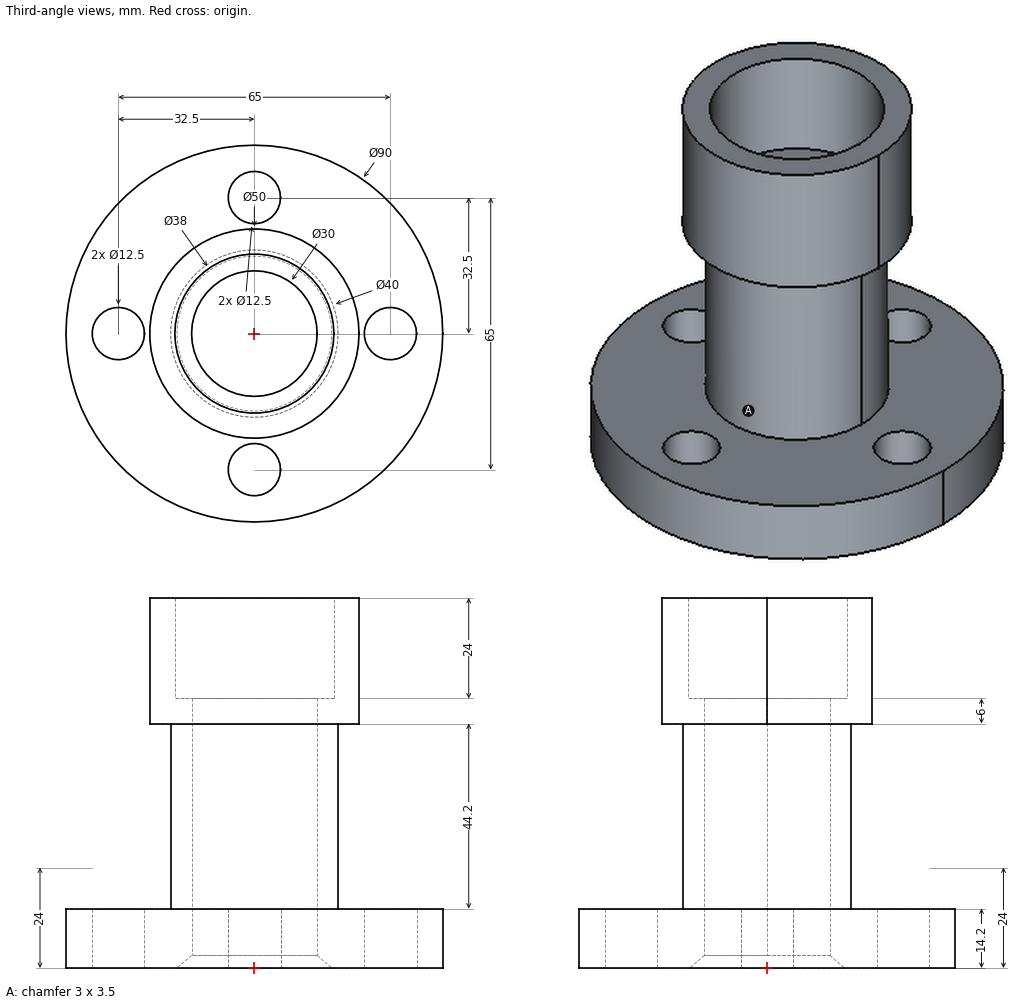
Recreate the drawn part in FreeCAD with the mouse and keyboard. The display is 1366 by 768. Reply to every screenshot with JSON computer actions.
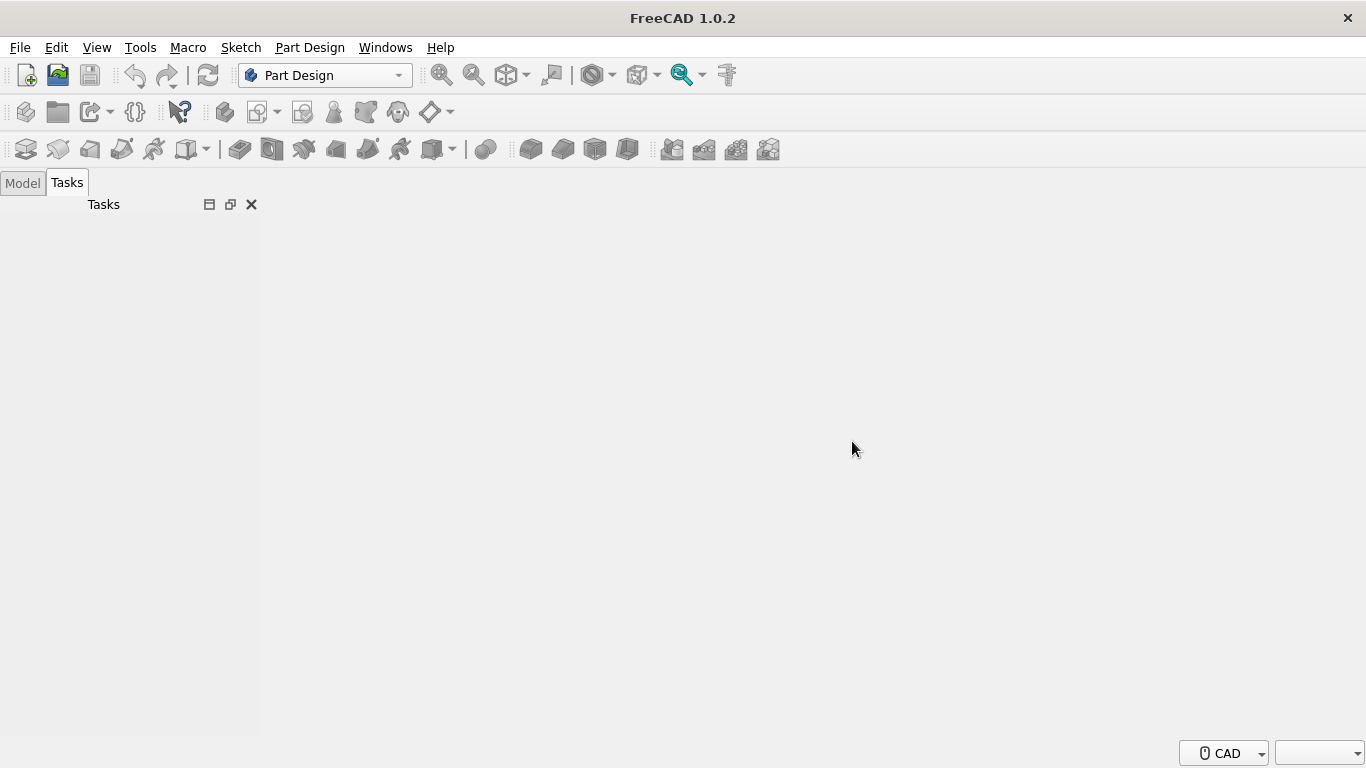
{"action": "left_click", "coordinate": [26, 76]}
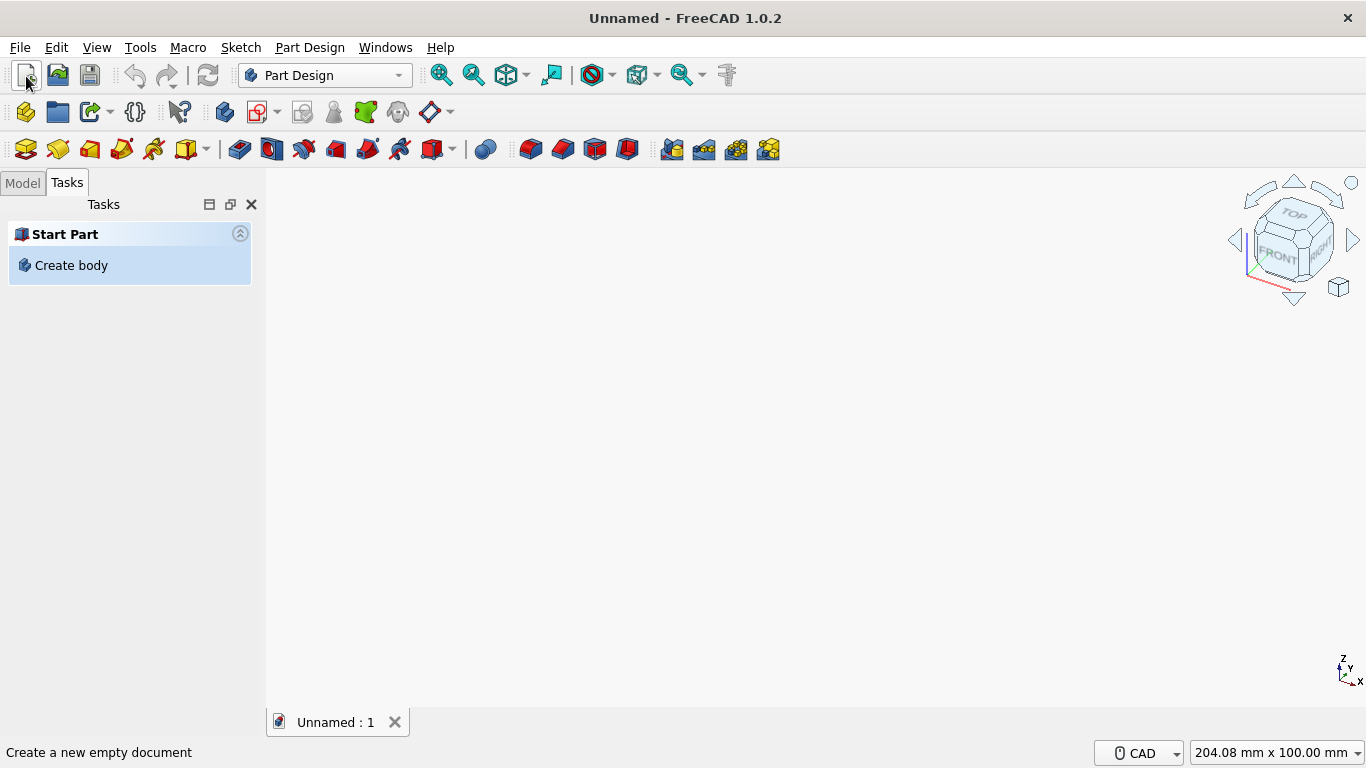
{"action": "left_click", "coordinate": [258, 112]}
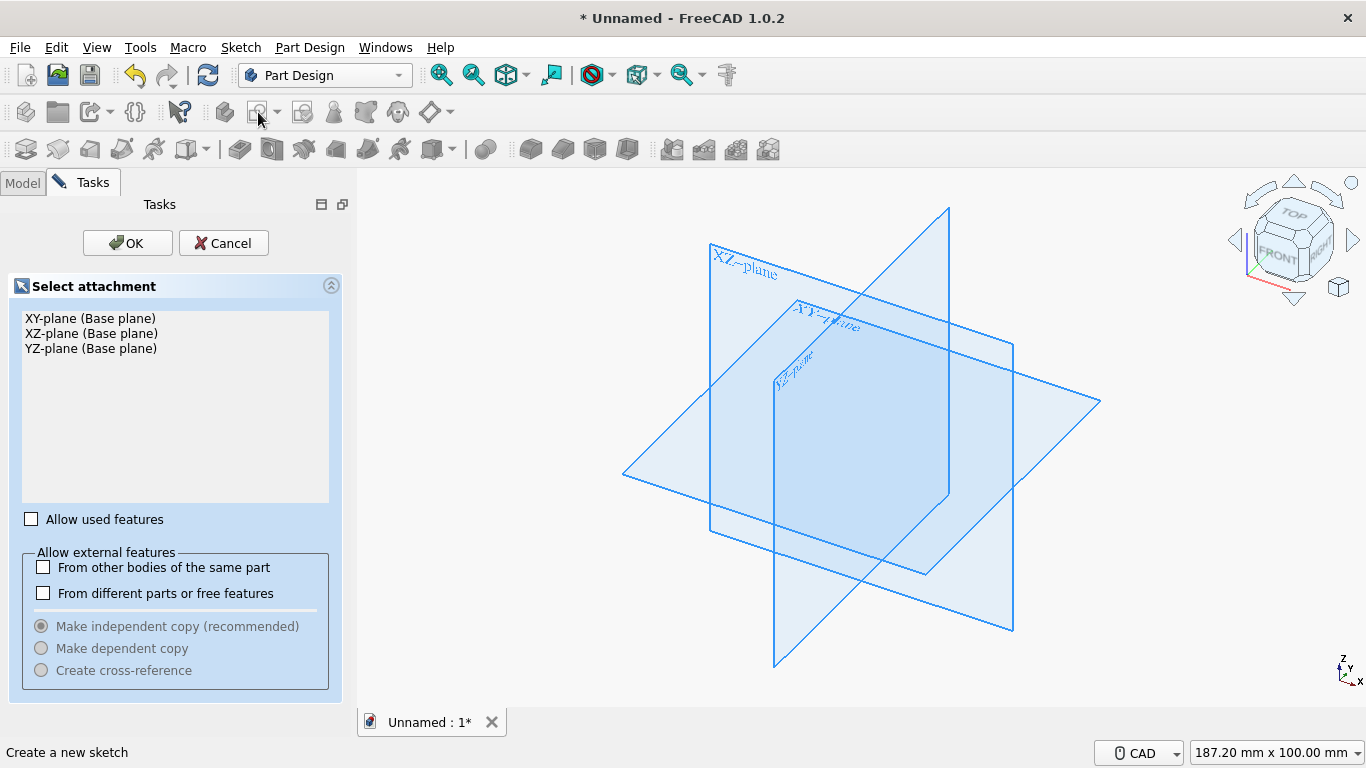
{"action": "left_click", "coordinate": [82, 318]}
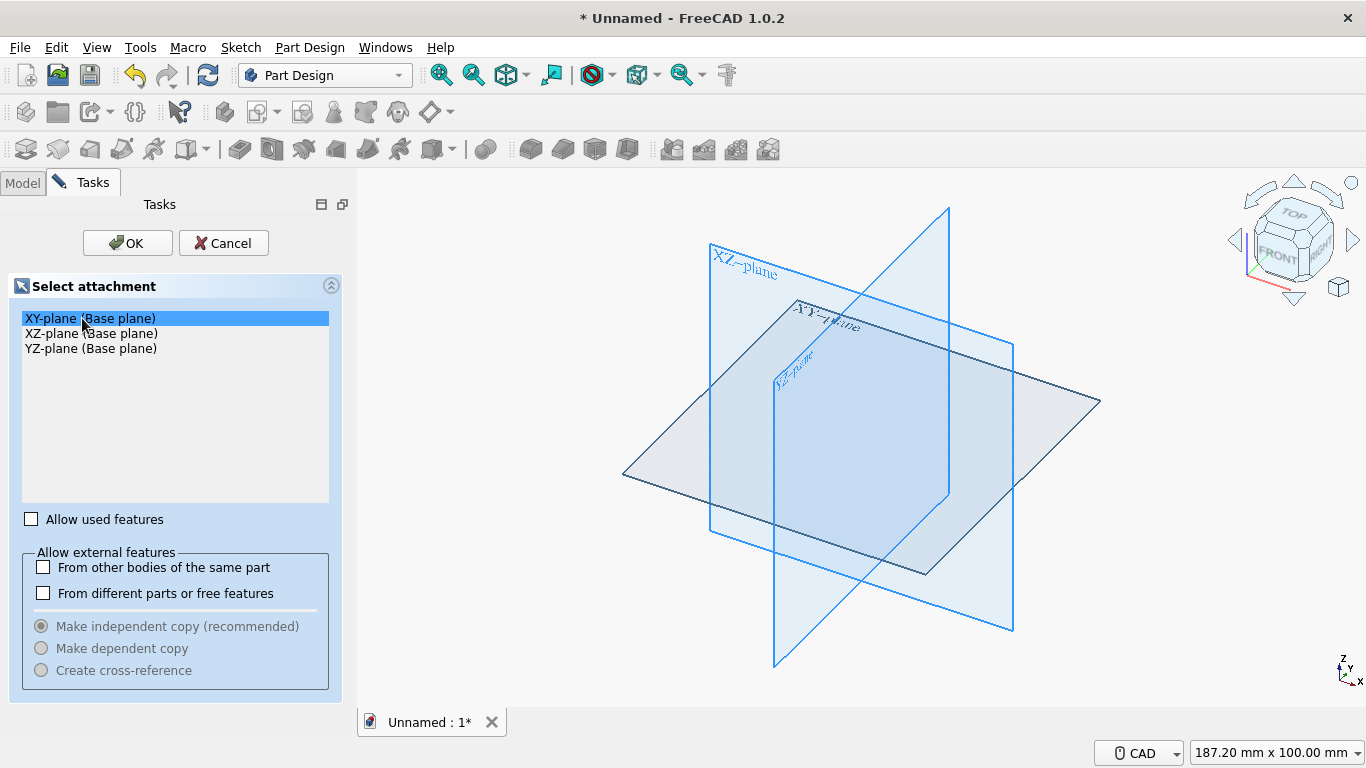
{"action": "left_click", "coordinate": [128, 243]}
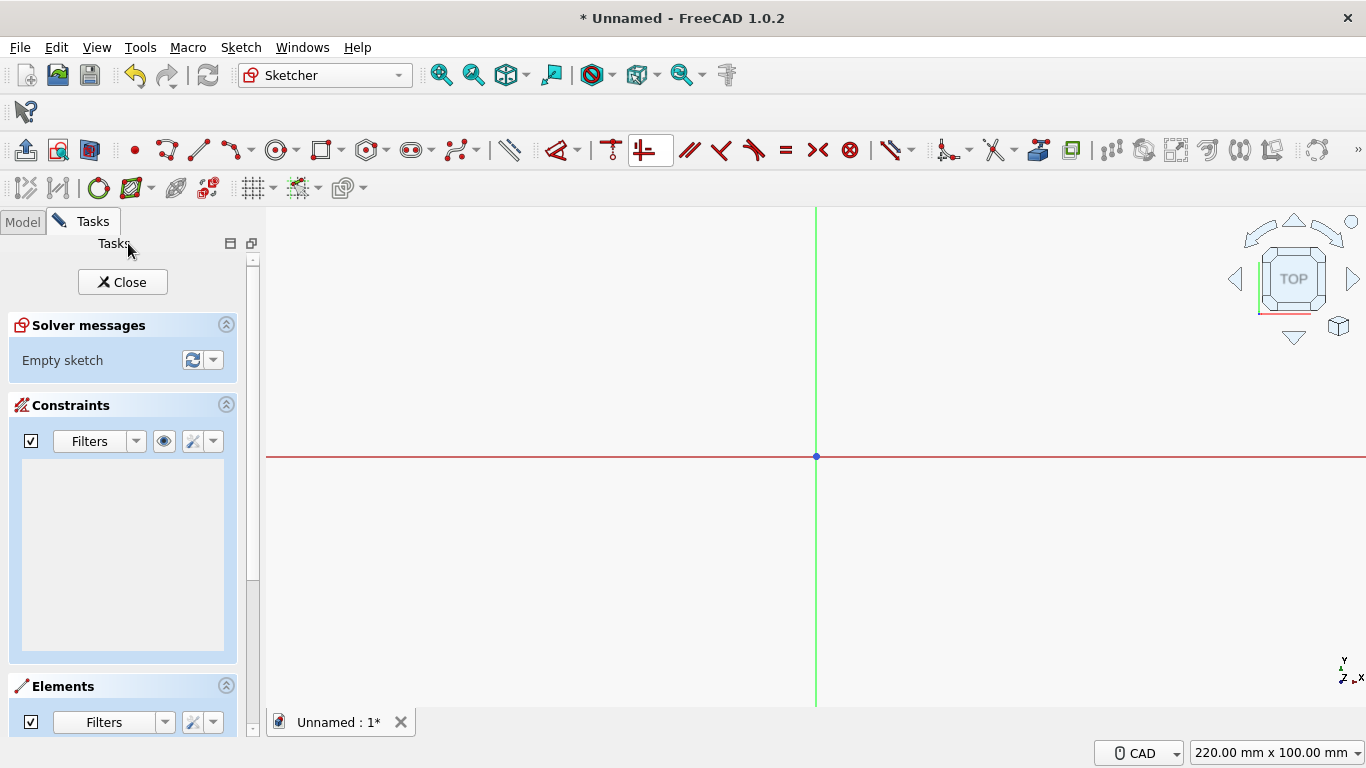
{"action": "scroll", "coordinate": [608, 457], "scroll_direction": "down", "scroll_amount": 2}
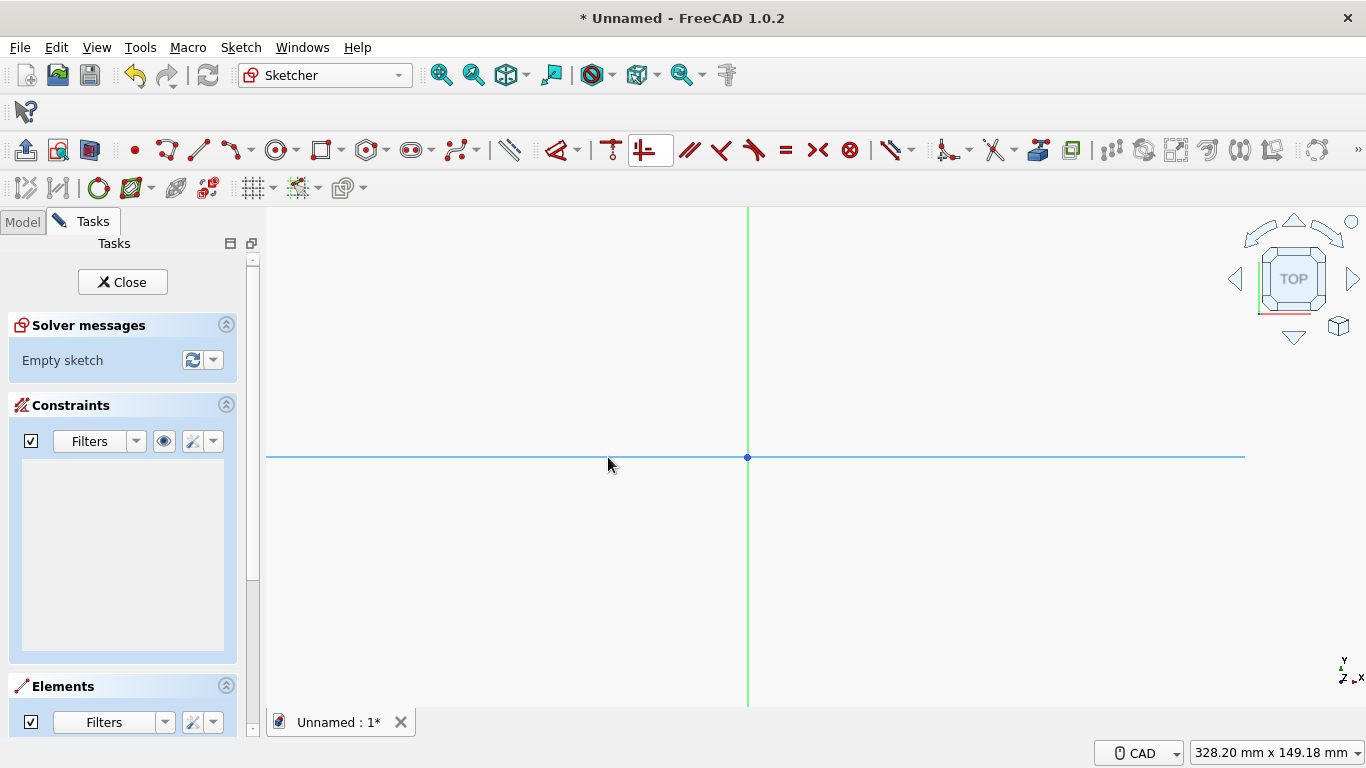
{"action": "left_click", "coordinate": [276, 150]}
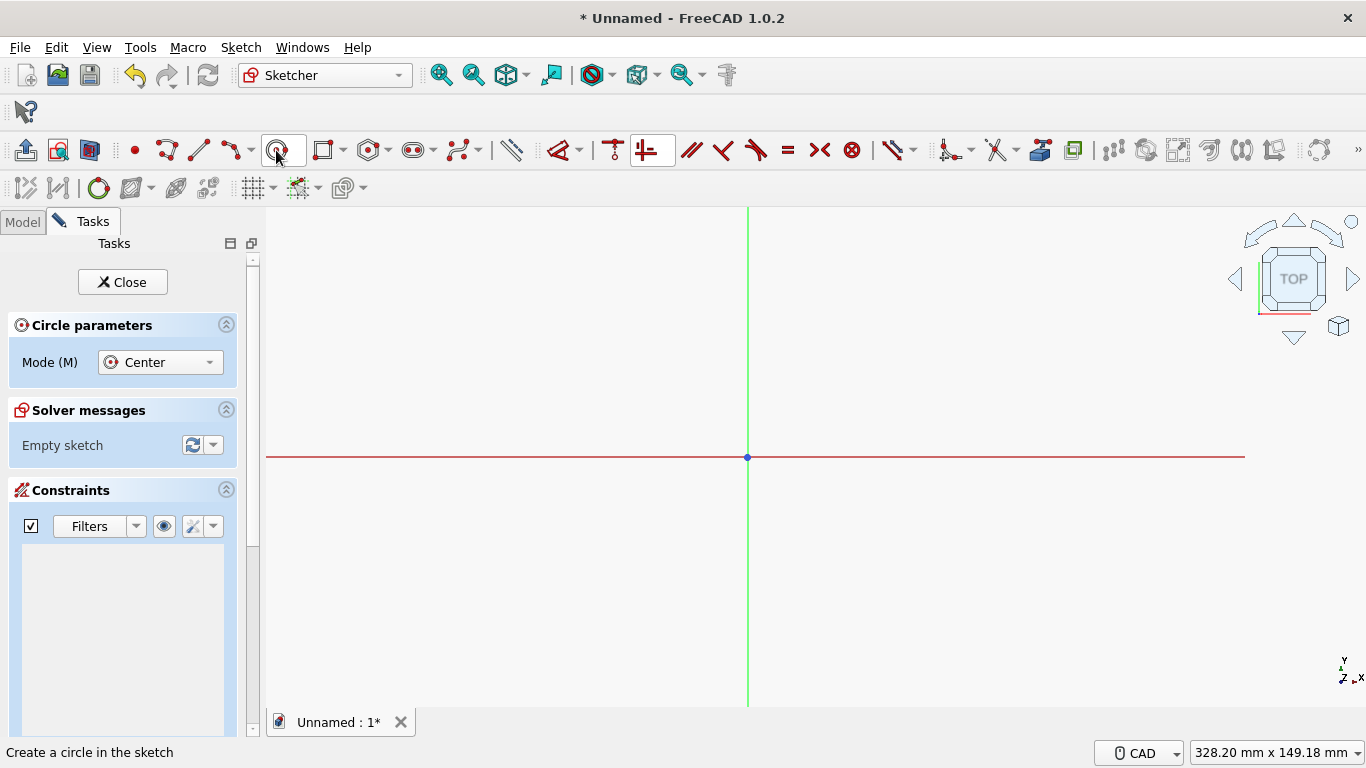
{"action": "left_click", "coordinate": [748, 457]}
{"action": "mouse_move", "coordinate": [854, 351]}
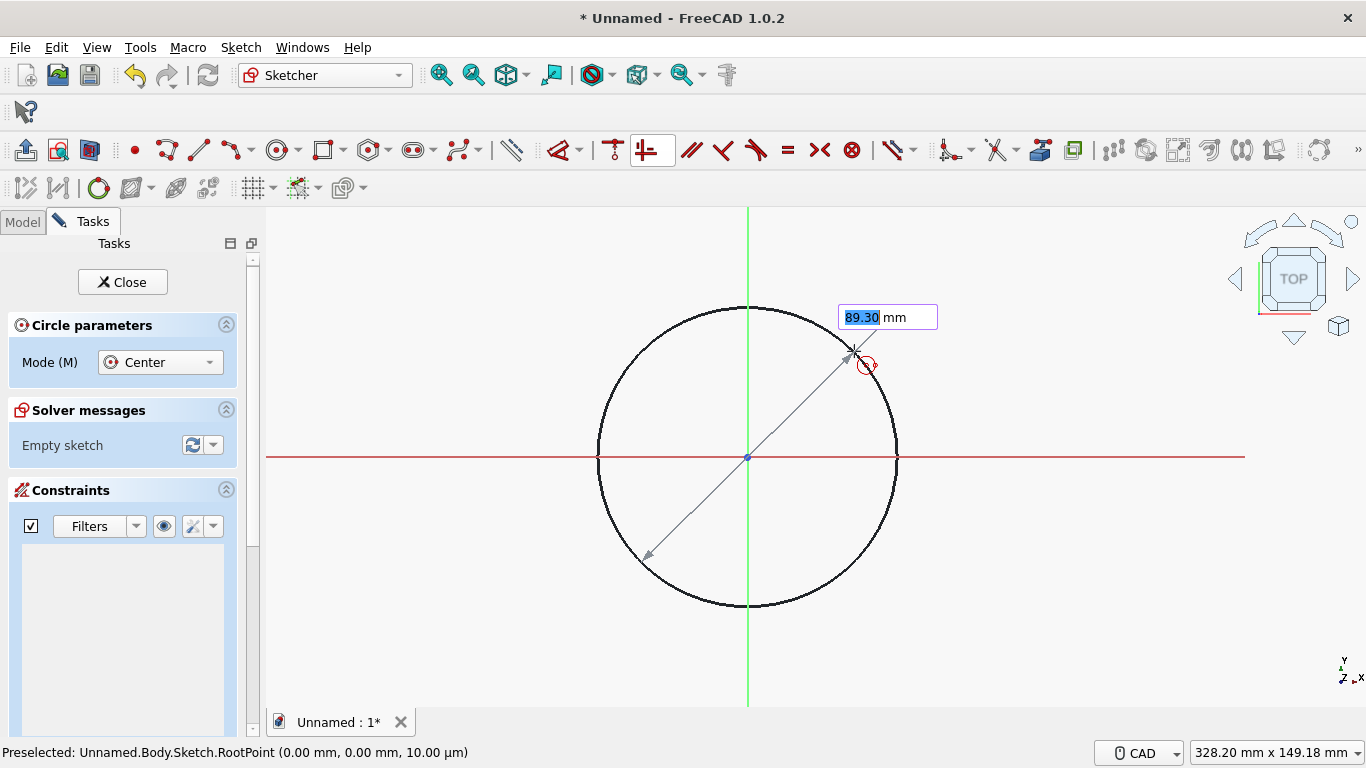
{"action": "type", "text": "90"}
{"action": "key", "text": "Return"}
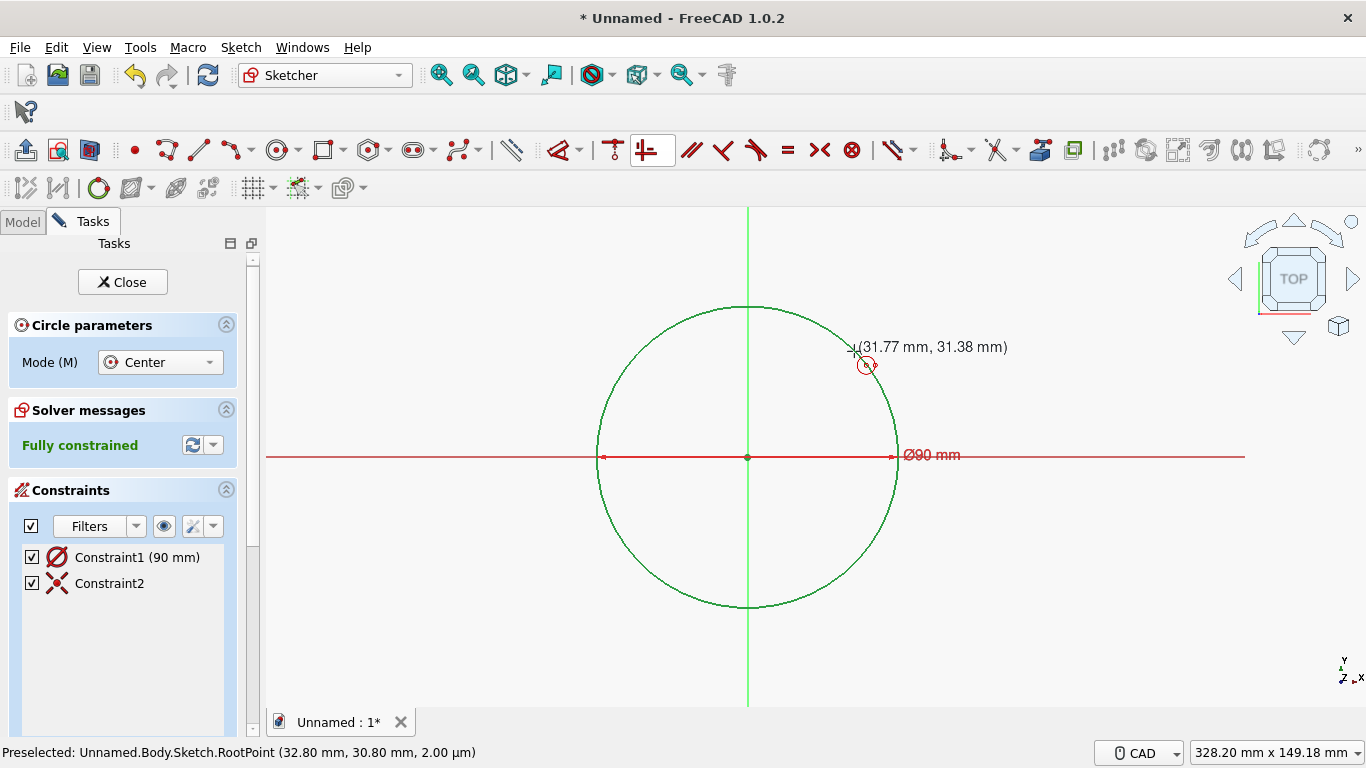
{"action": "left_click", "coordinate": [748, 457]}
{"action": "mouse_move", "coordinate": [783, 422]}